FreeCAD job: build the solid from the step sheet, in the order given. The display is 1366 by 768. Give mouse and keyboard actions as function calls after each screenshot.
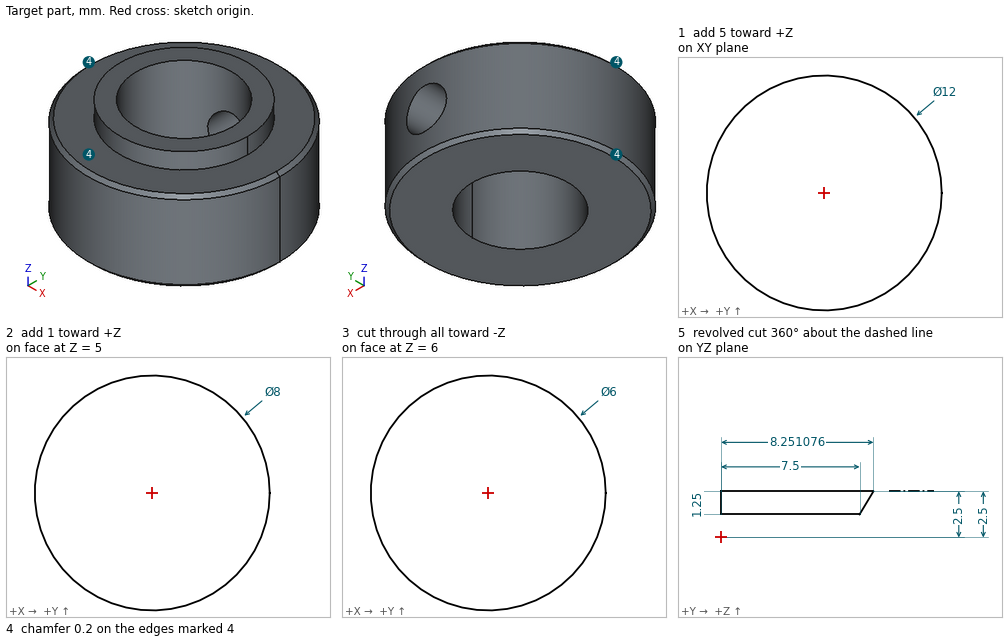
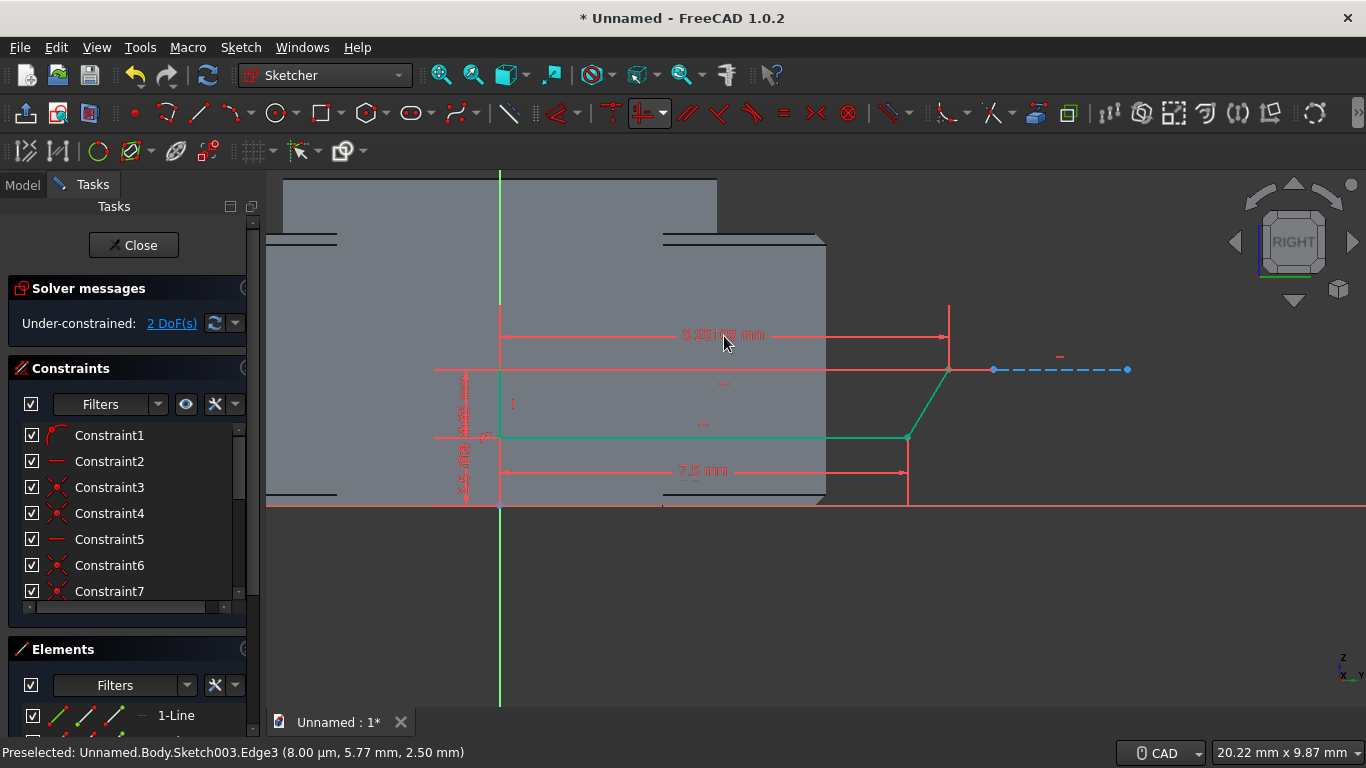
click(134, 245)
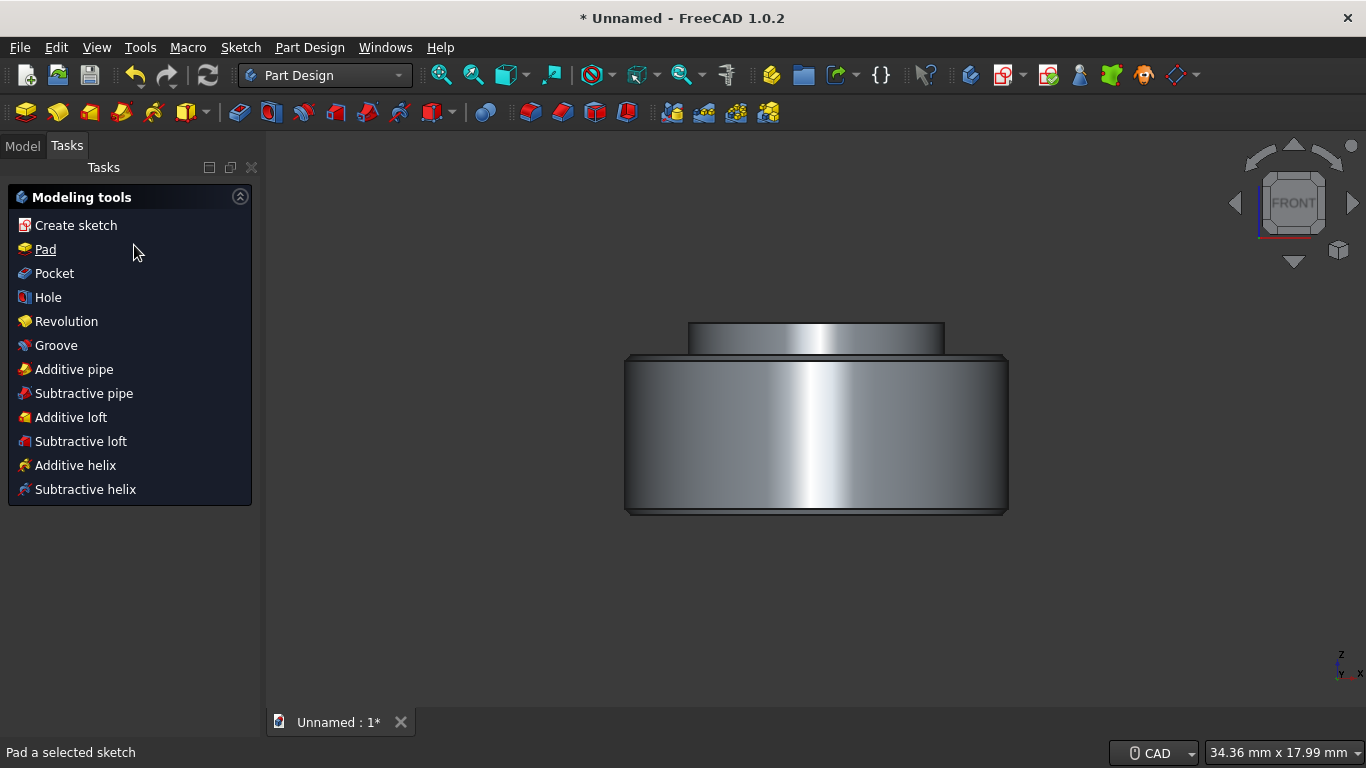
click(304, 112)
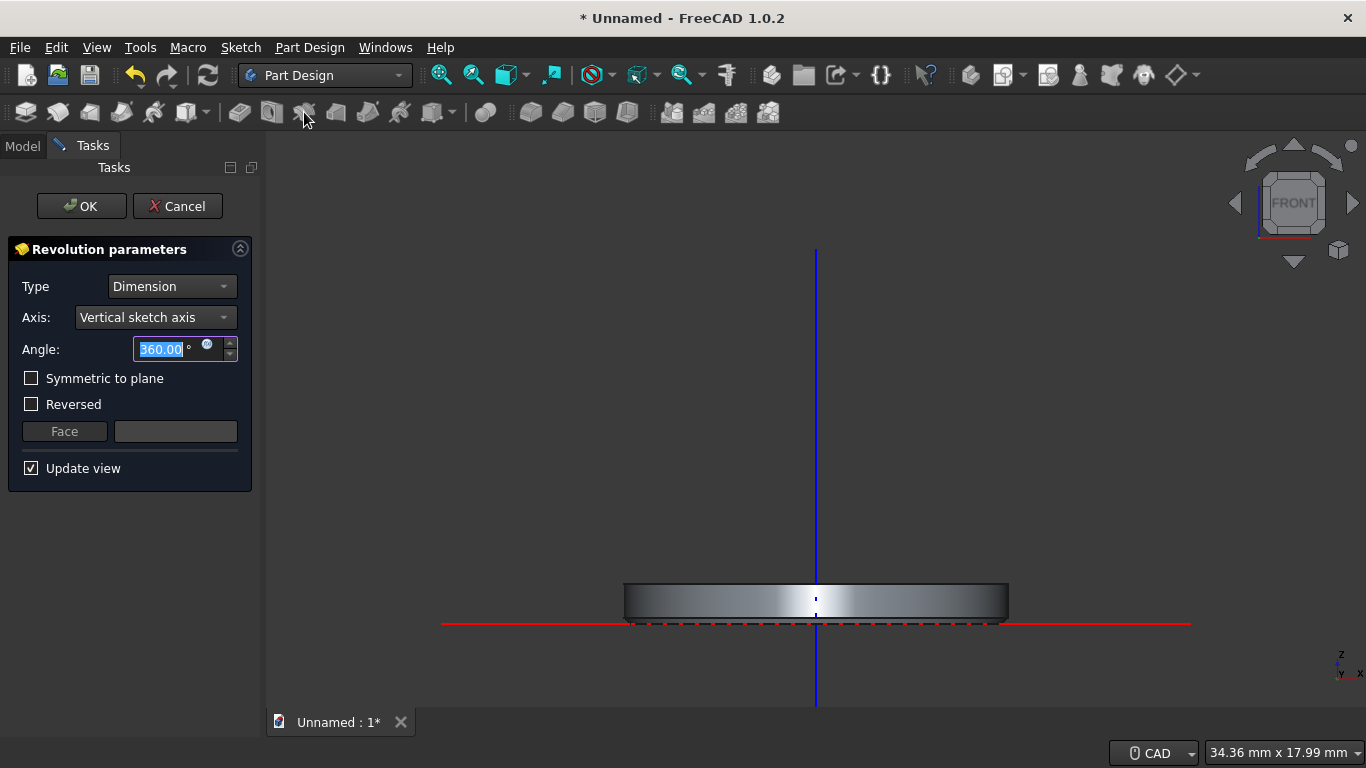
click(156, 318)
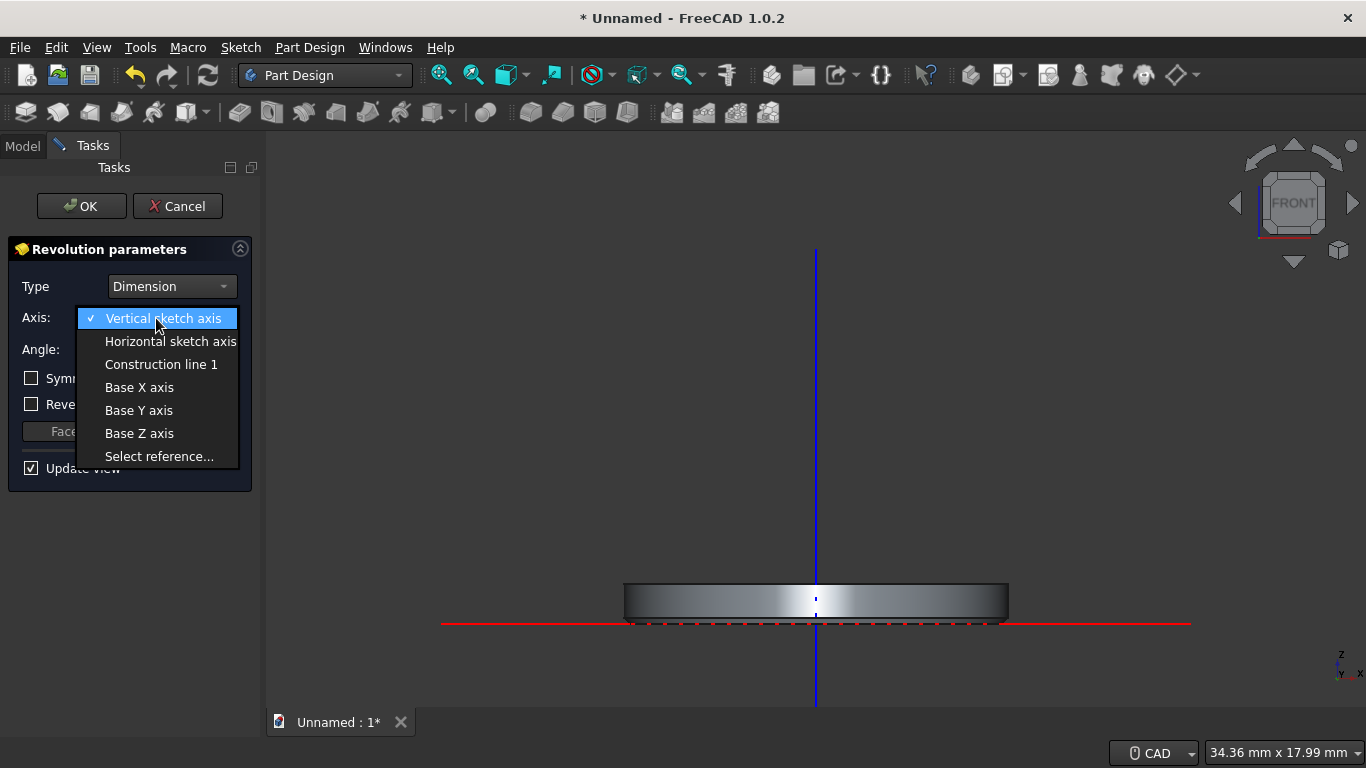
click(156, 364)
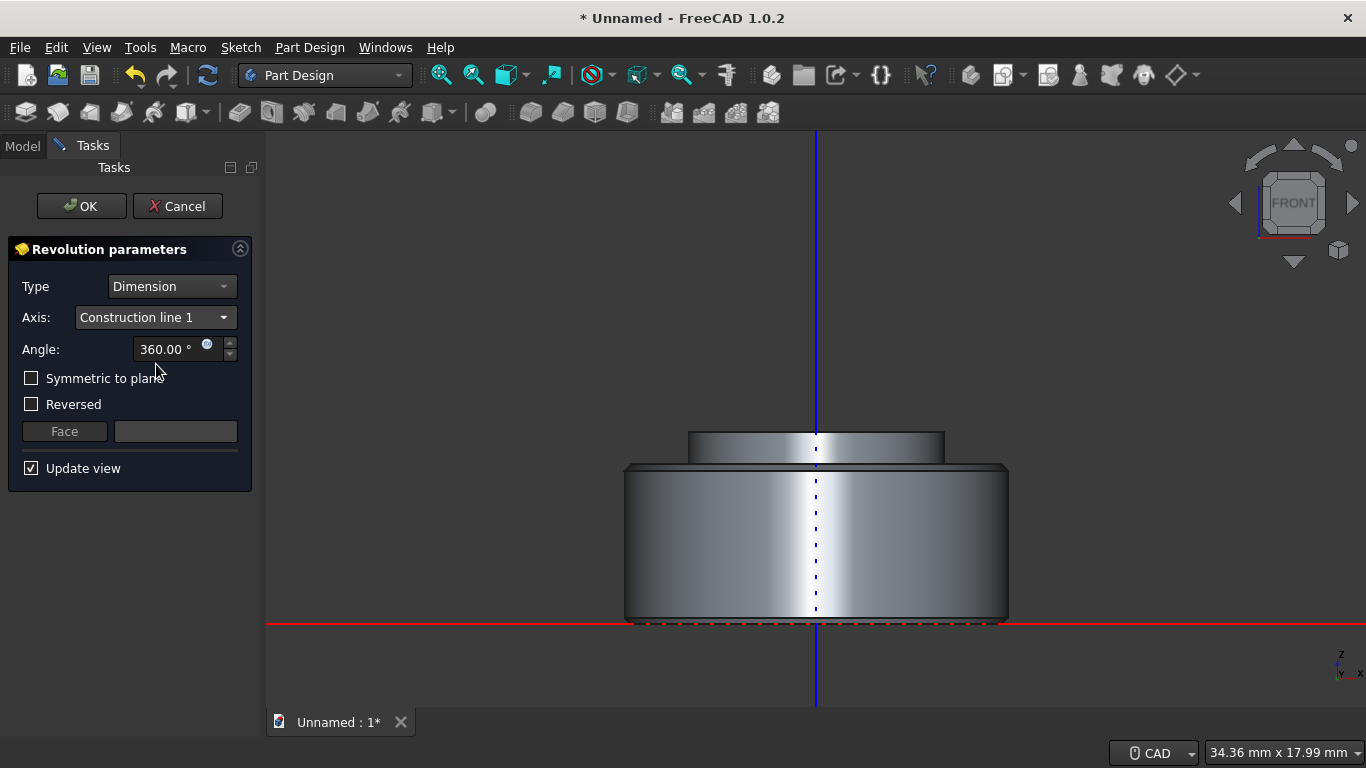
click(82, 206)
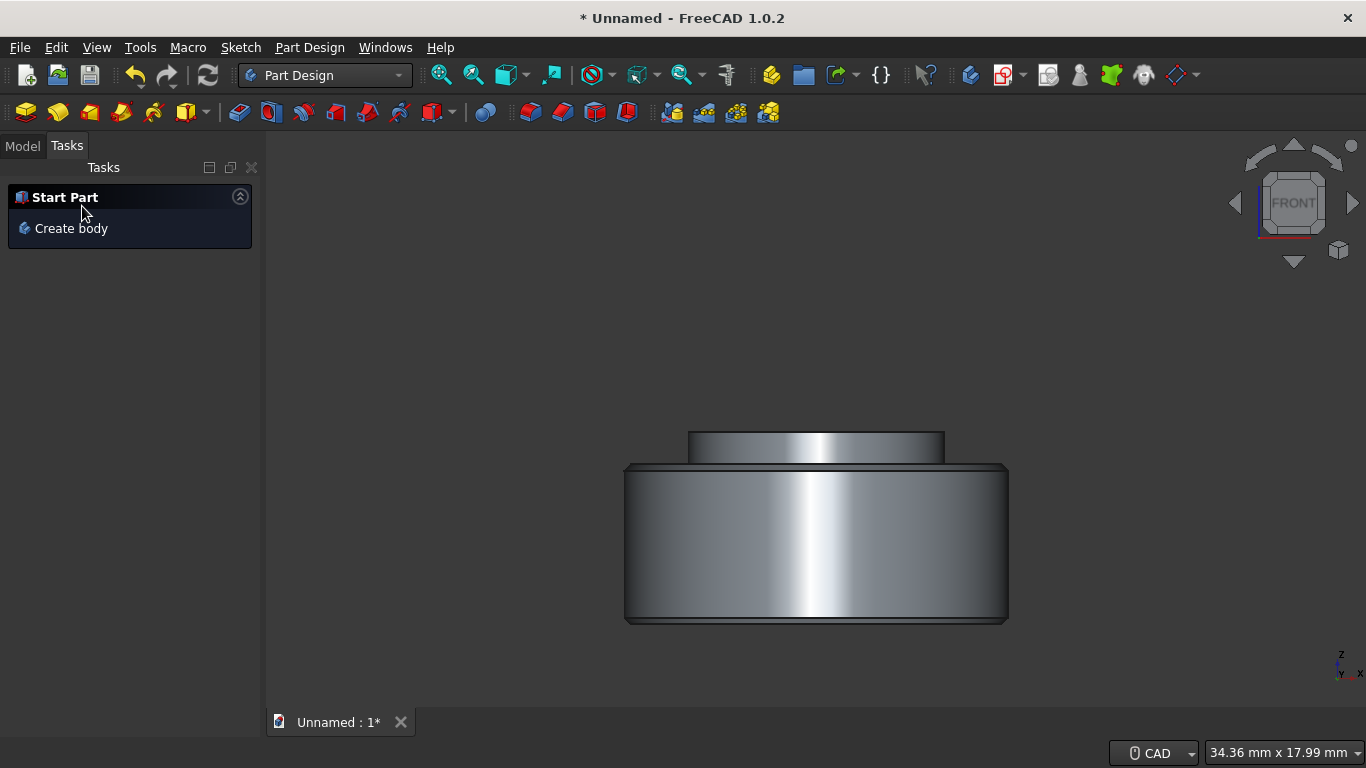
key(0)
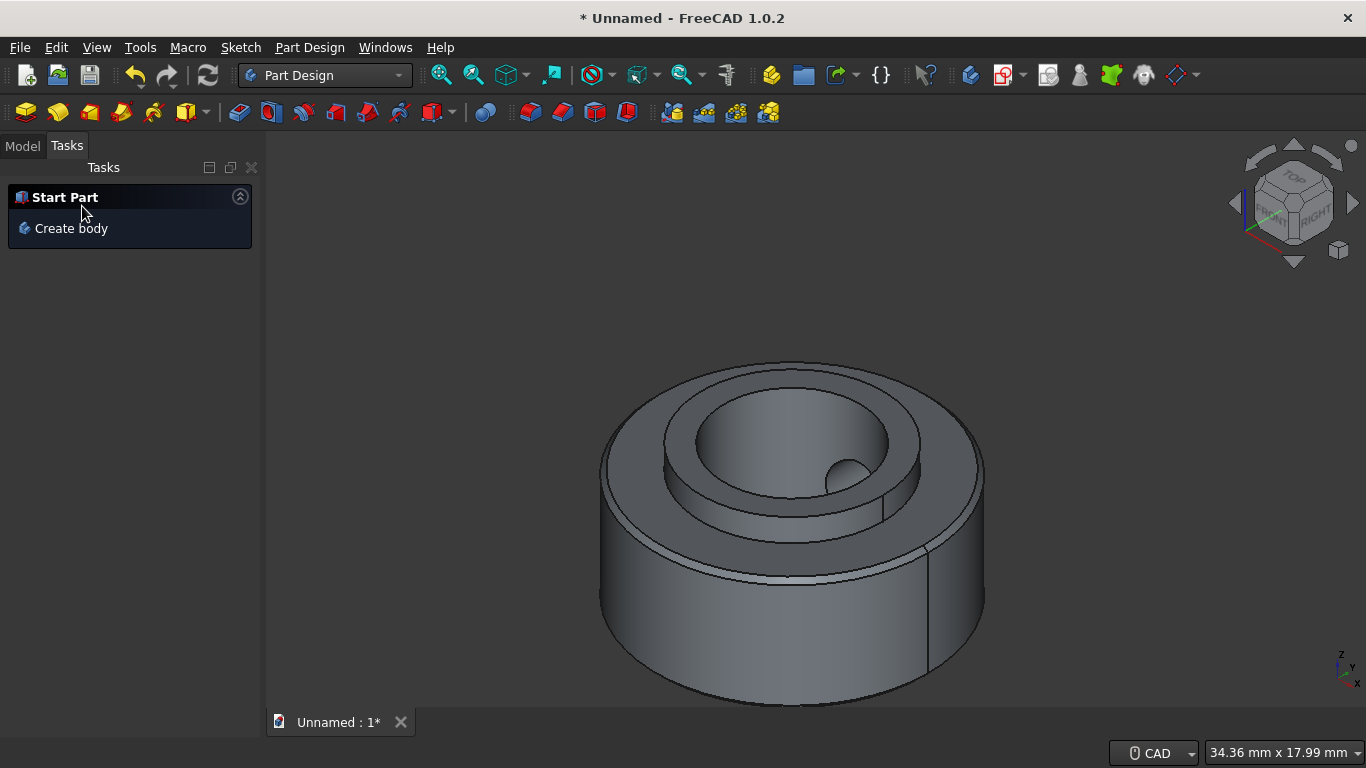
key(v)
key(f)